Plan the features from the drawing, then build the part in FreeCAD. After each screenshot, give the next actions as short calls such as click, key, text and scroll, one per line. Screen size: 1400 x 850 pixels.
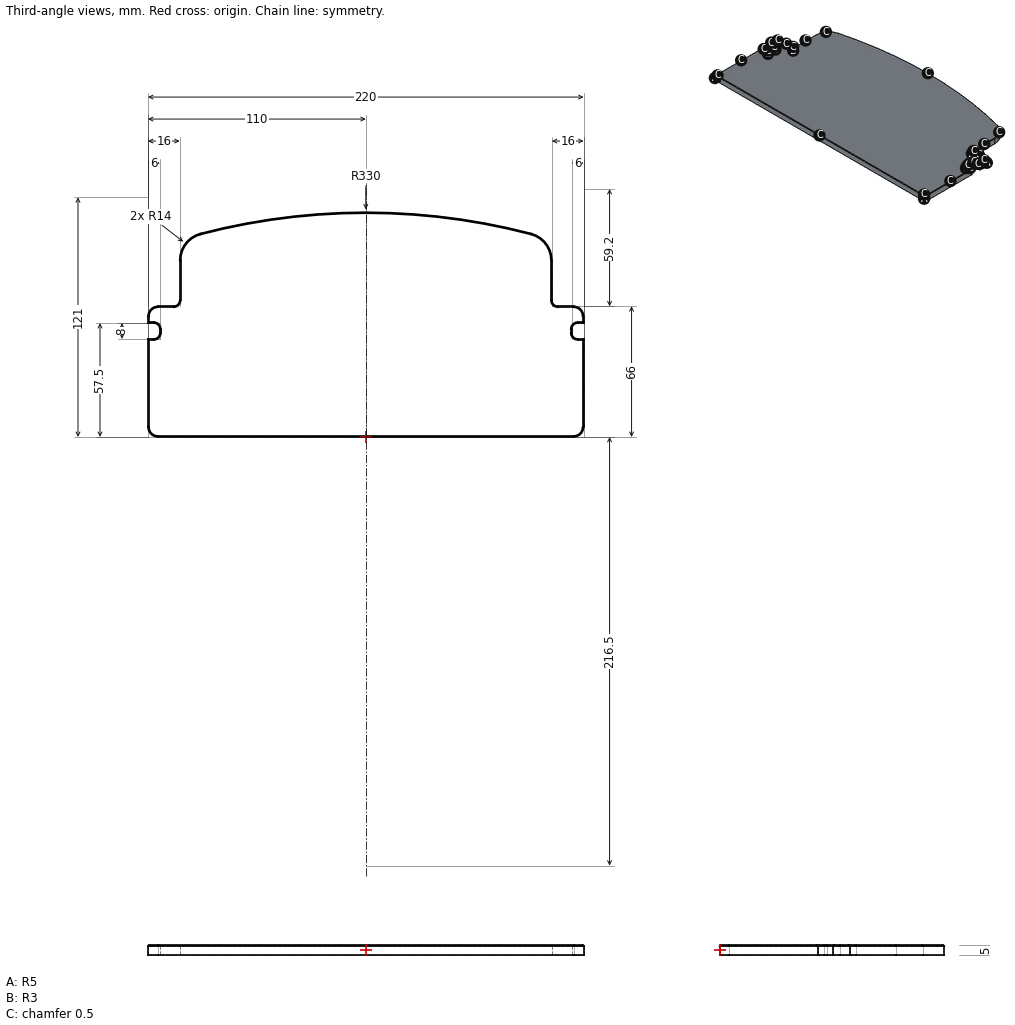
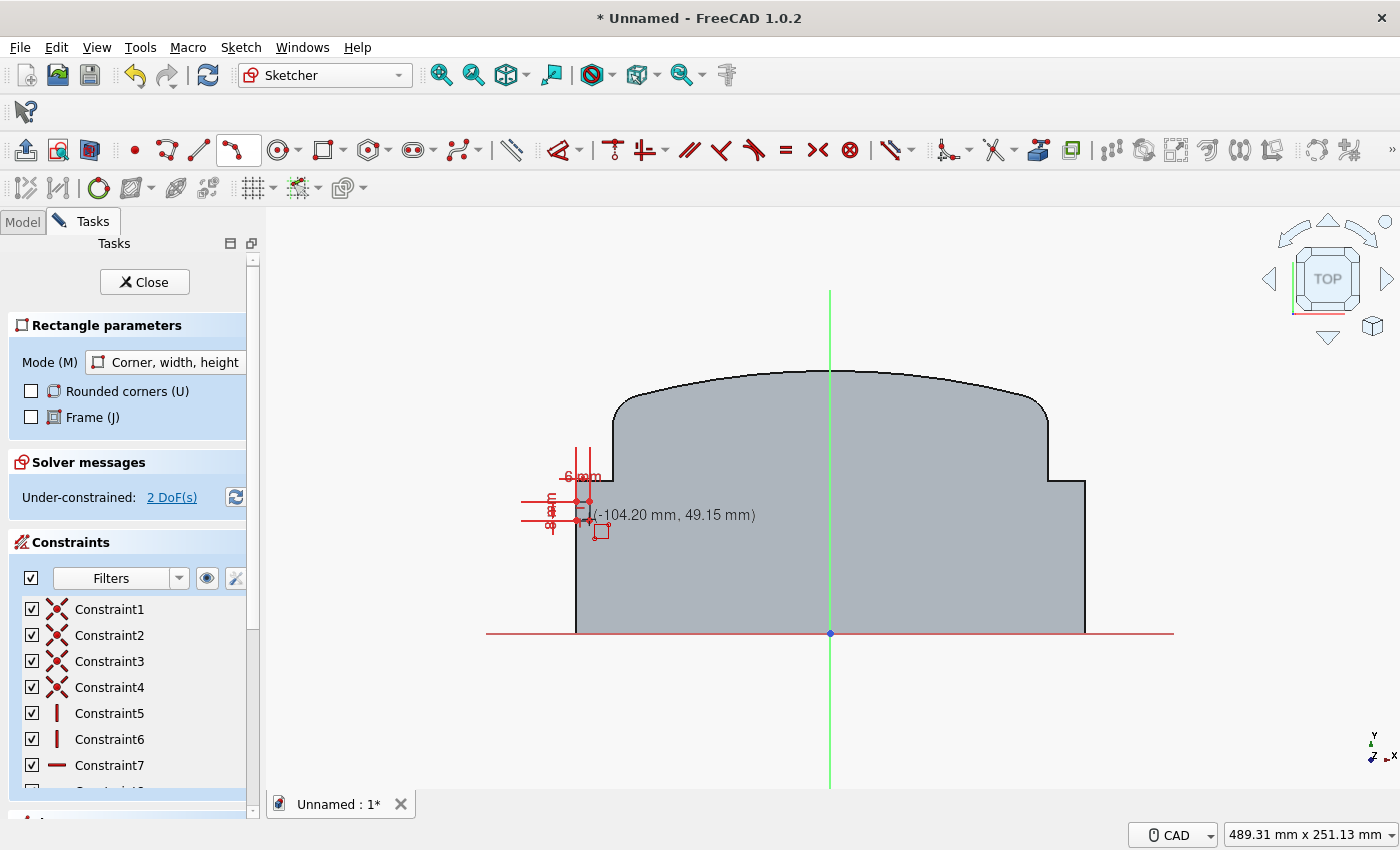
click(1072, 501)
move(1085, 519)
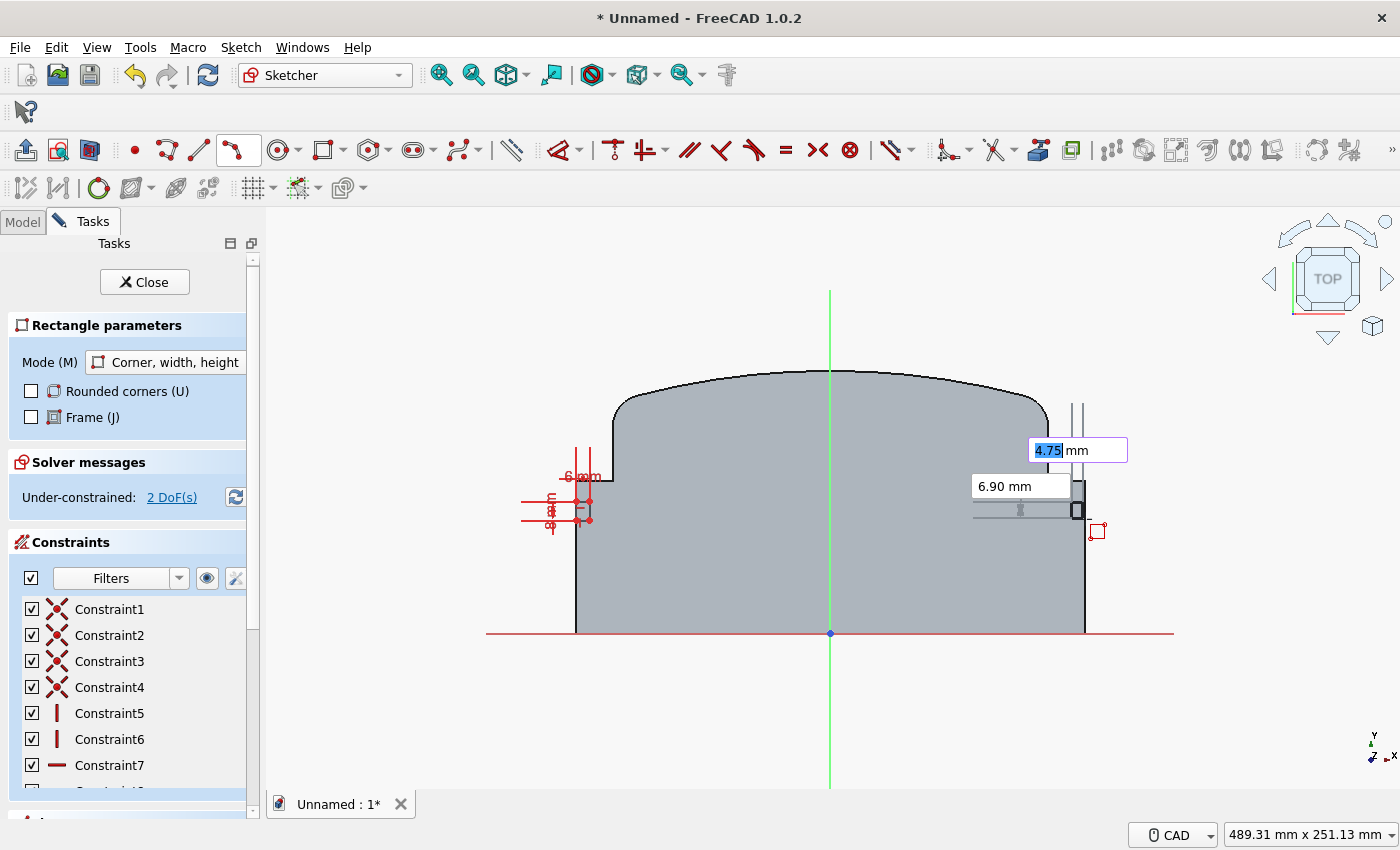
text(6)
key(Tab)
text(8)
key(Return)
key(Escape)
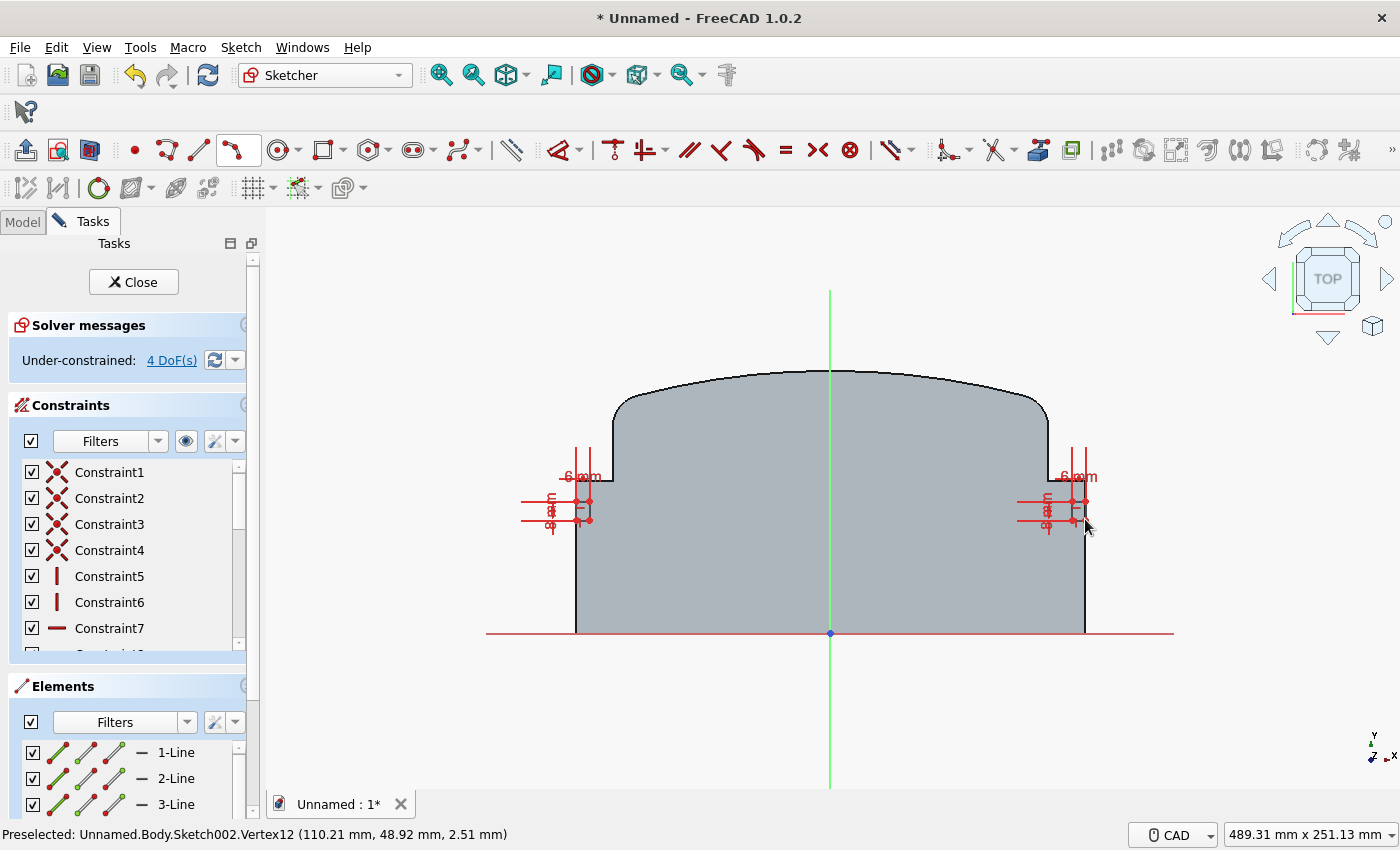
click(590, 502)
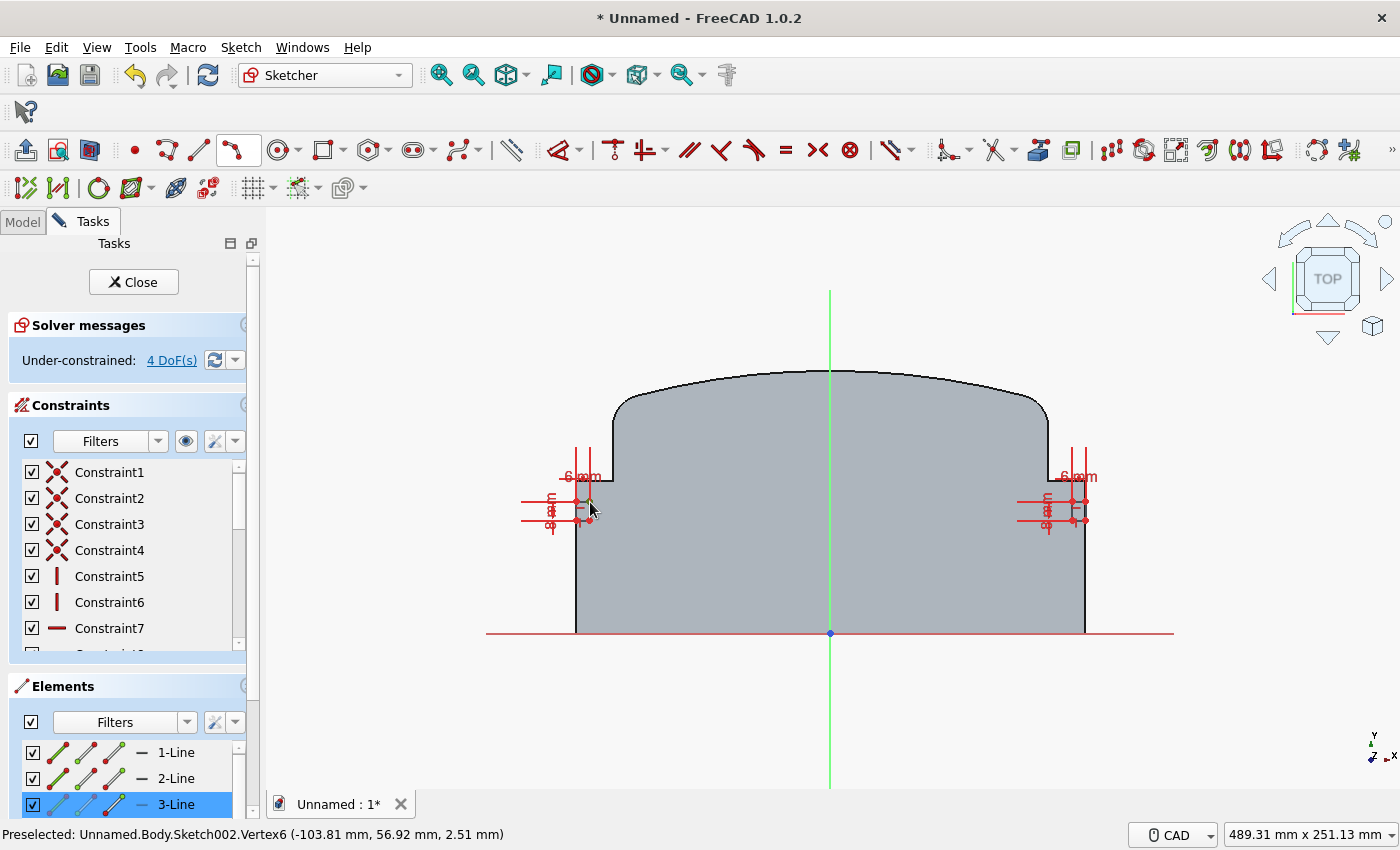
click(1072, 502)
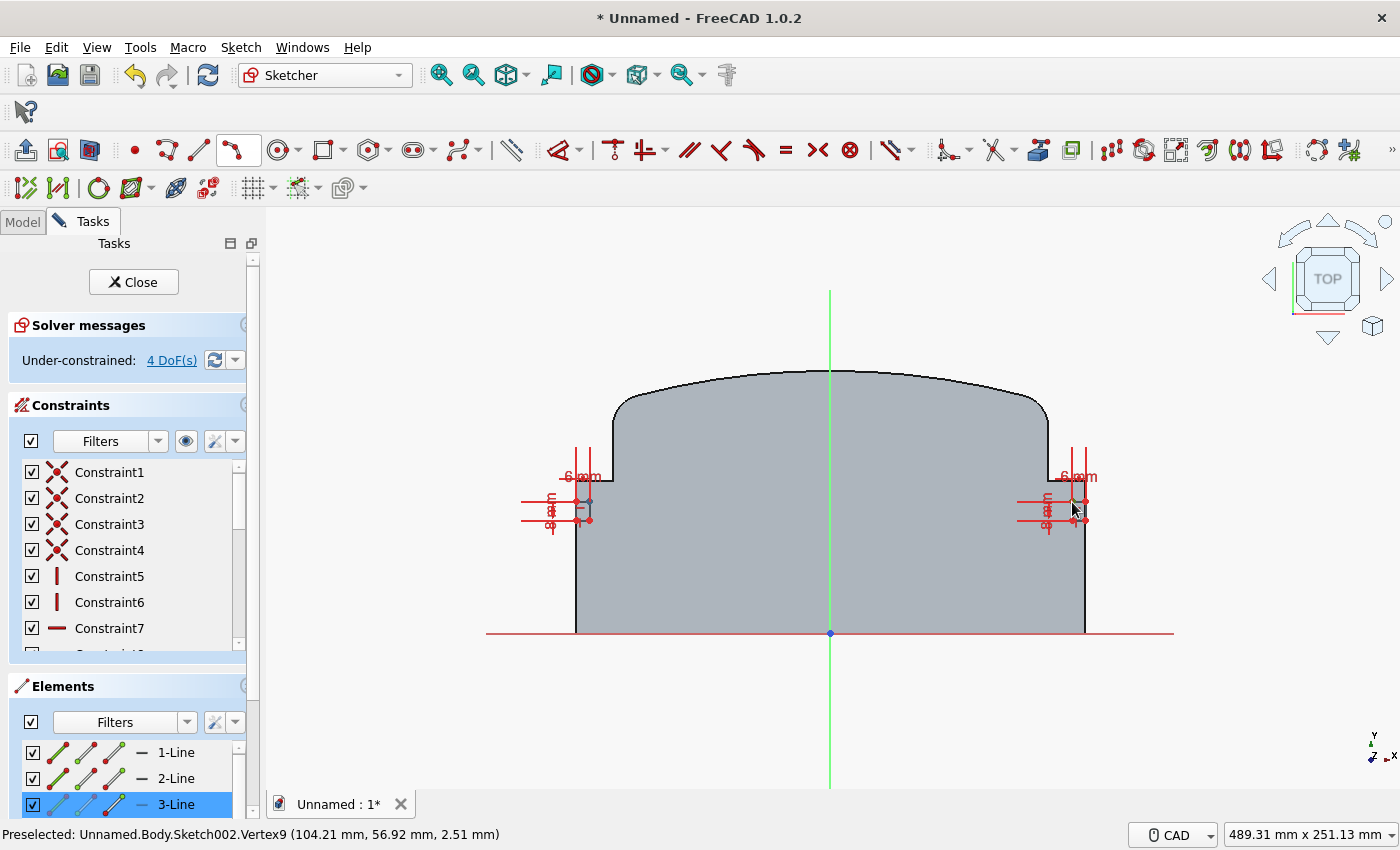
click(830, 723)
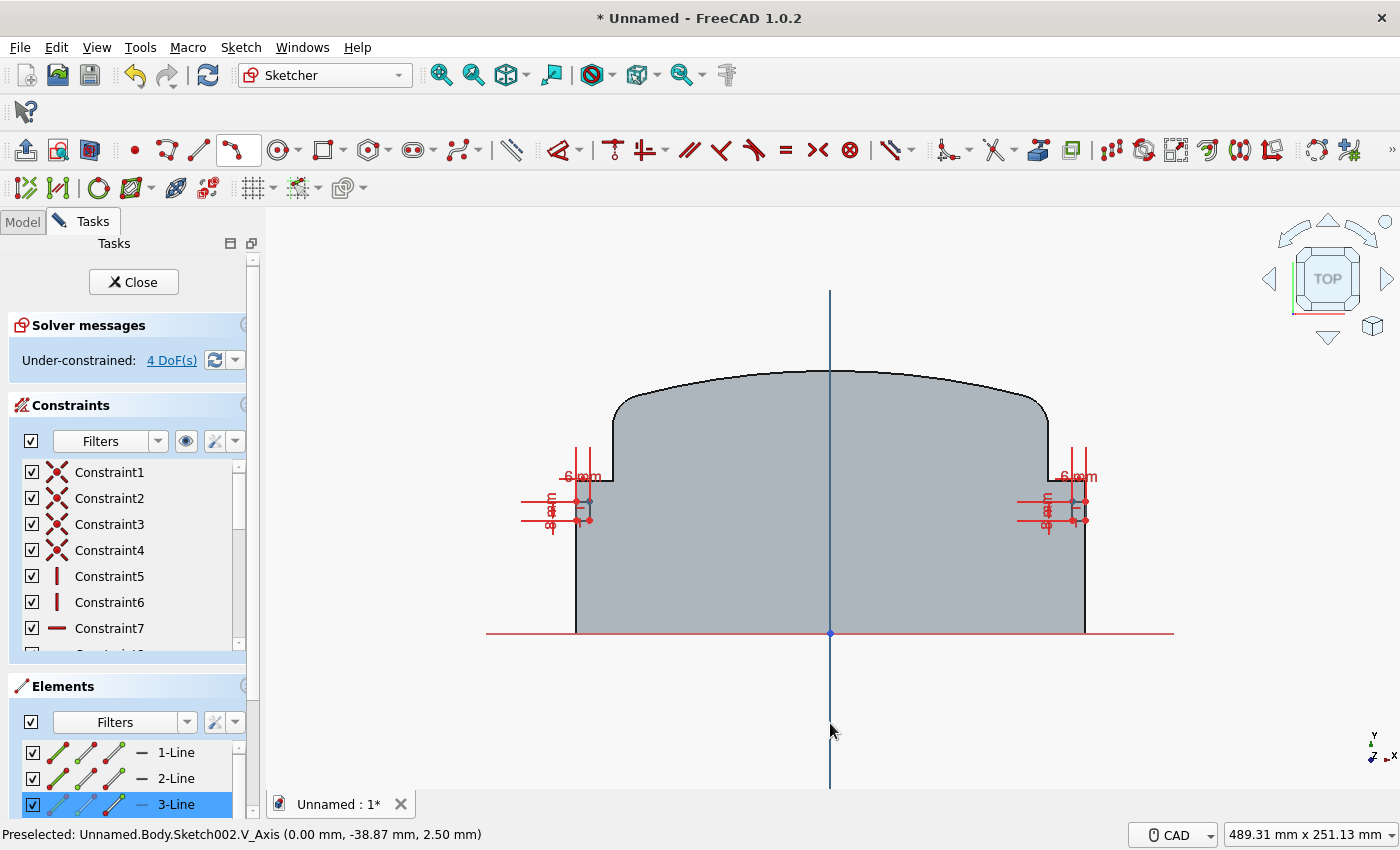
key(s)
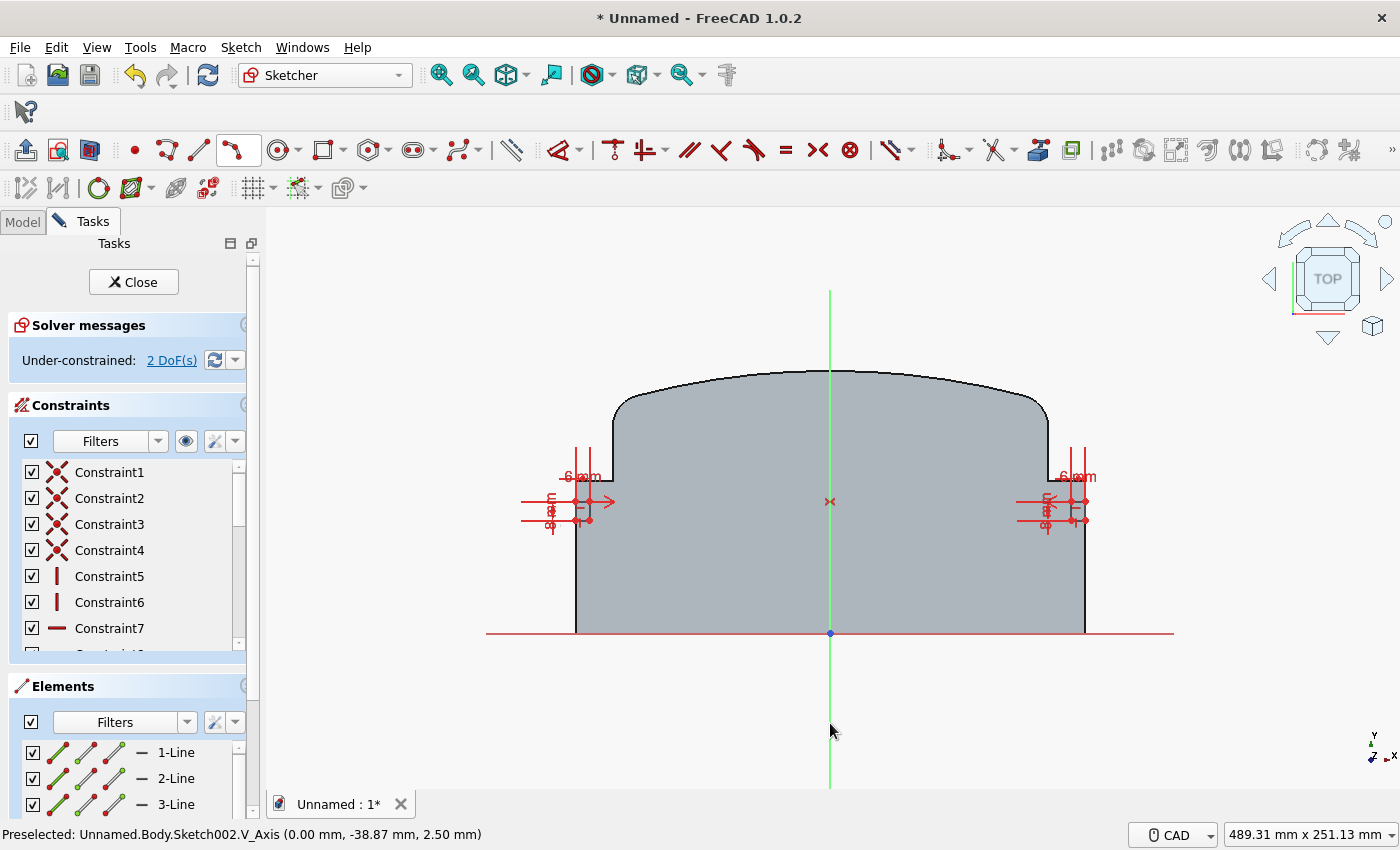
key(d)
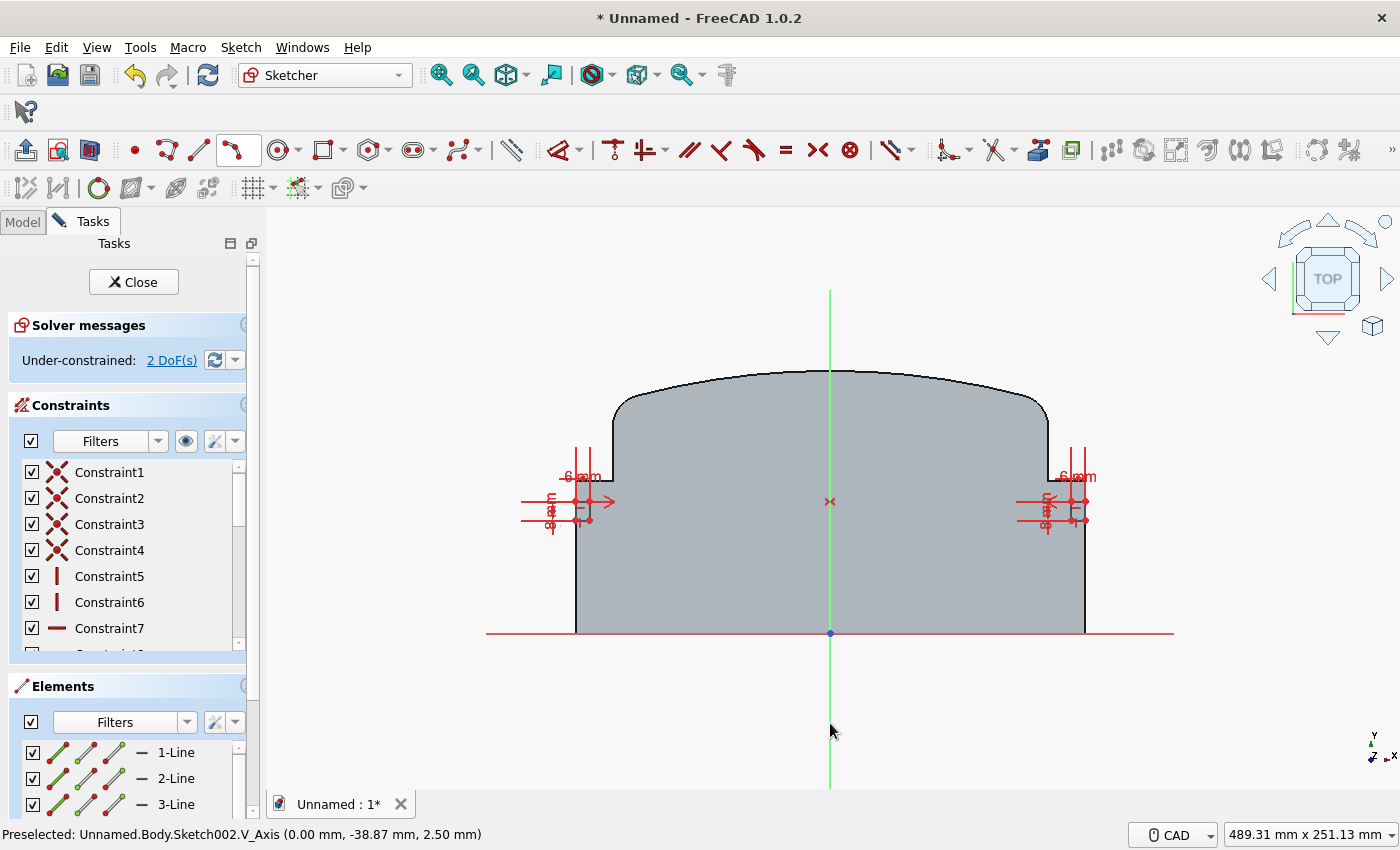
click(576, 502)
click(703, 668)